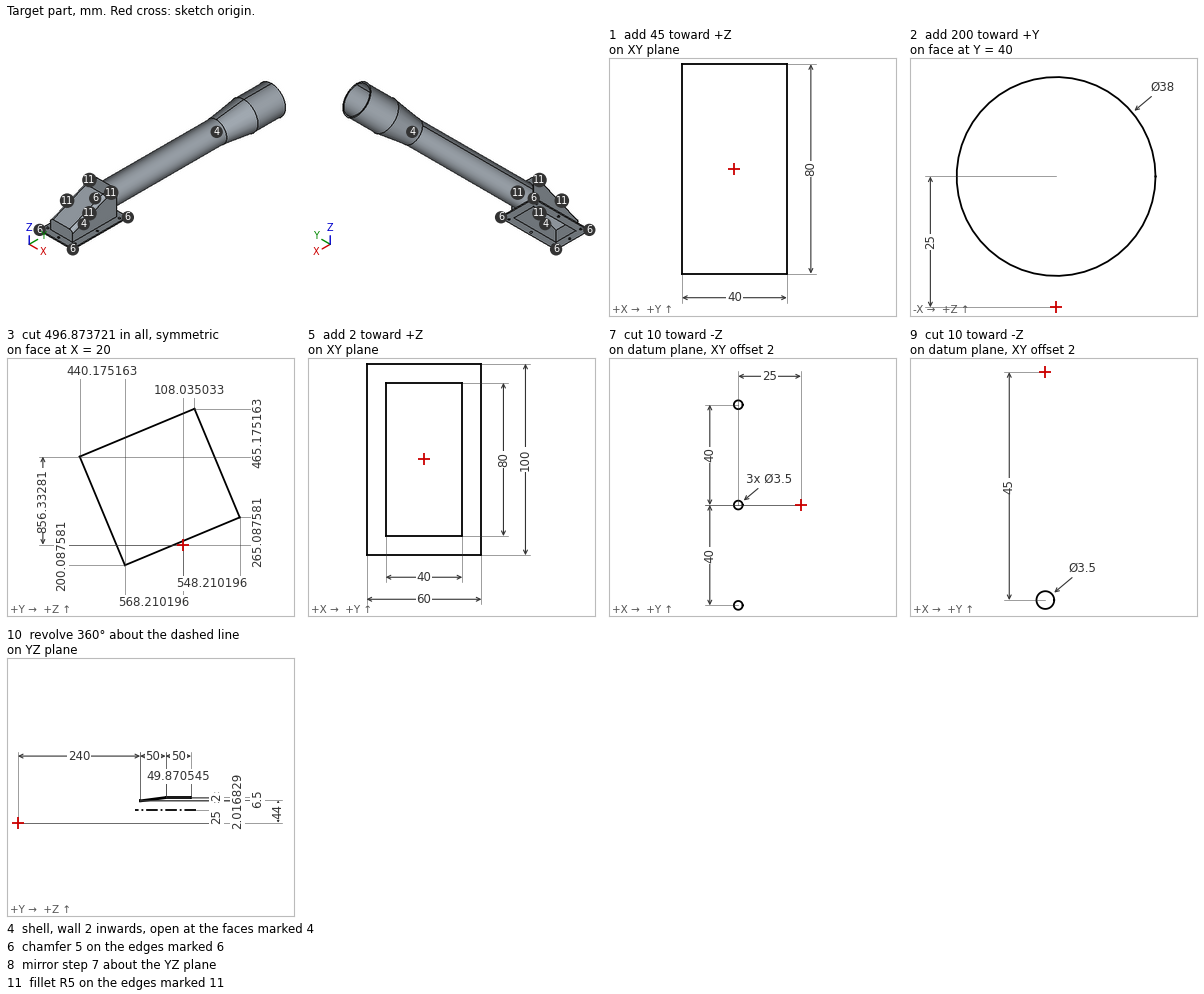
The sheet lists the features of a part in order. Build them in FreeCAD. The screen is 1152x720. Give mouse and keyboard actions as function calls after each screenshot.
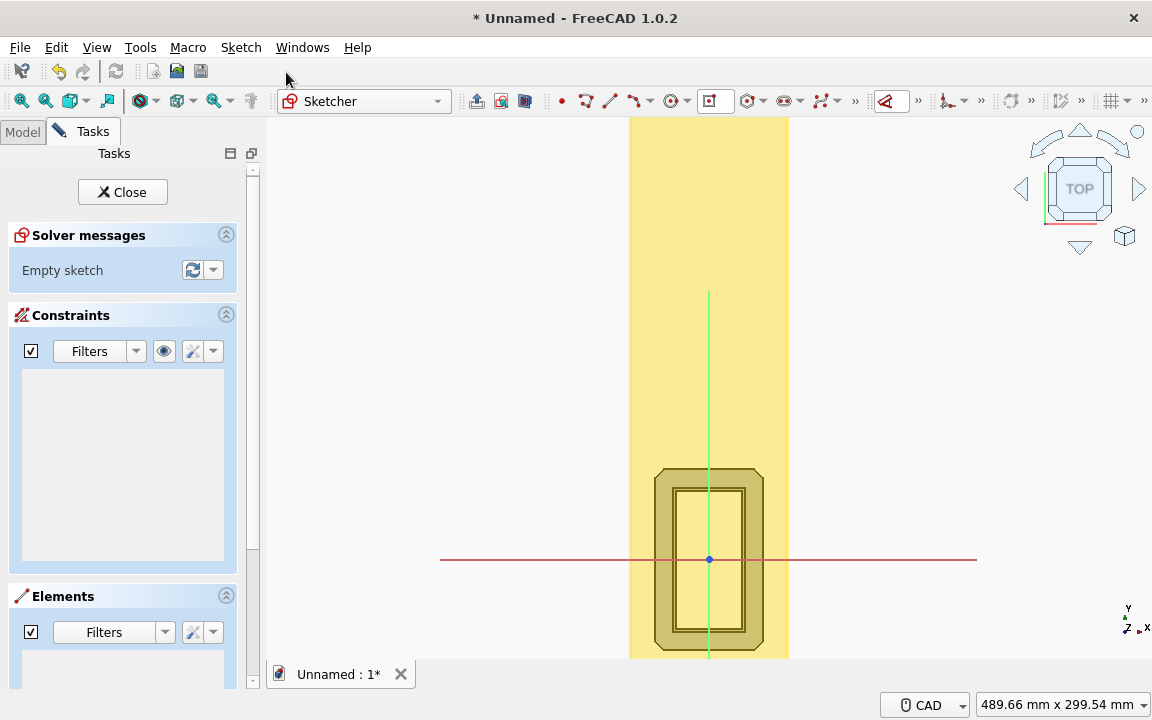
scroll(640, 388, down, 5)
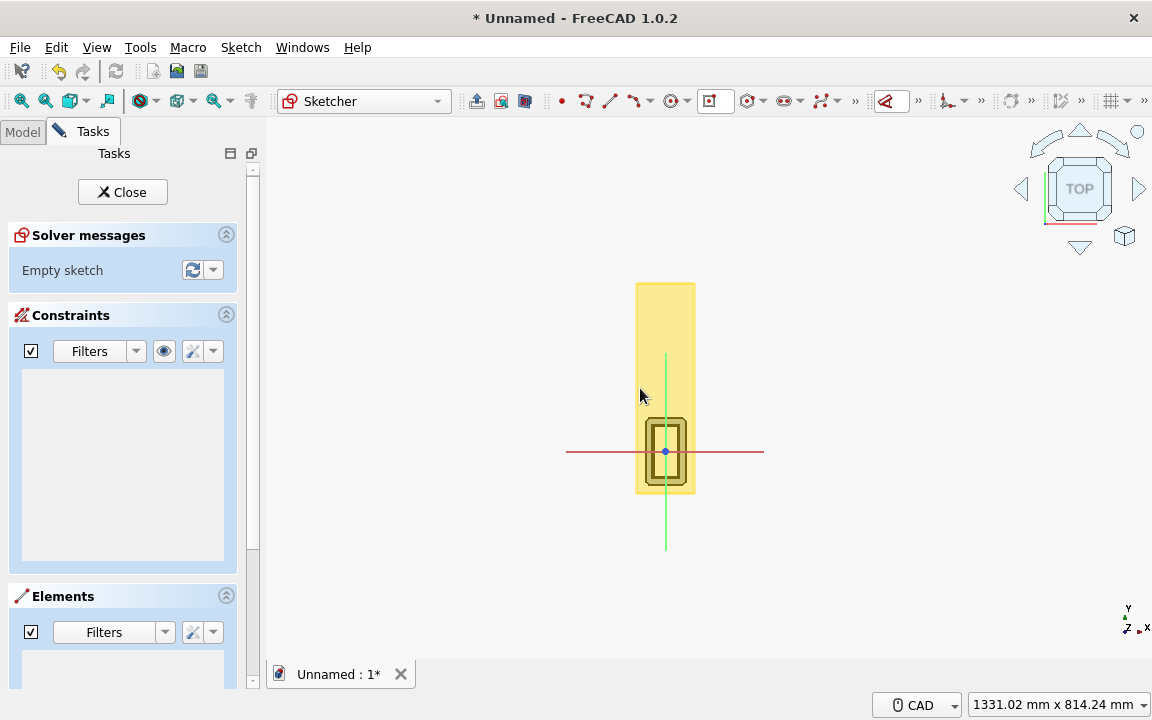
scroll(660, 464, up, 9)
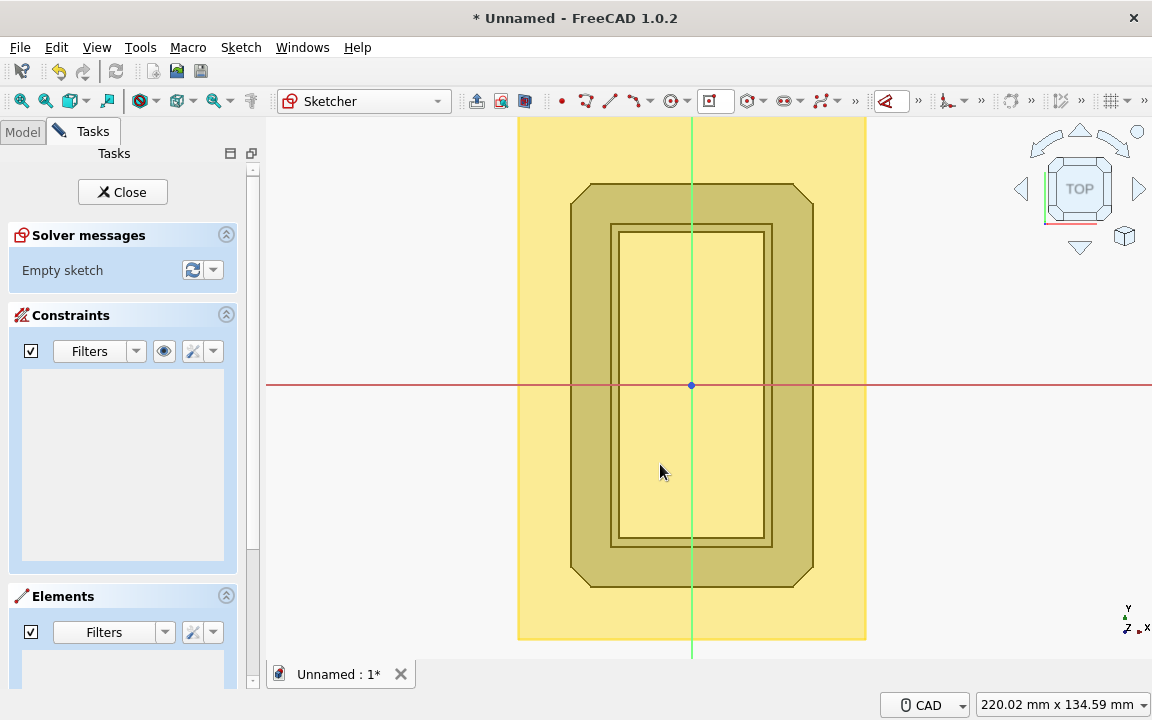
key(g)
key(c)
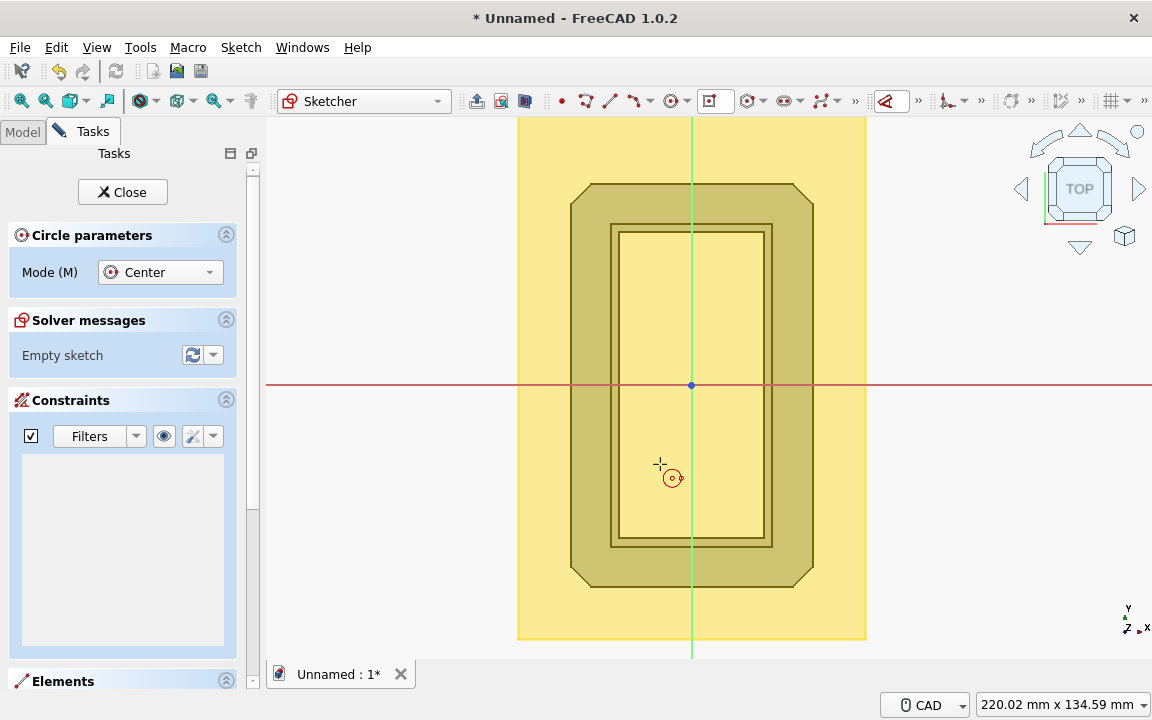
scroll(591, 385, up, 6)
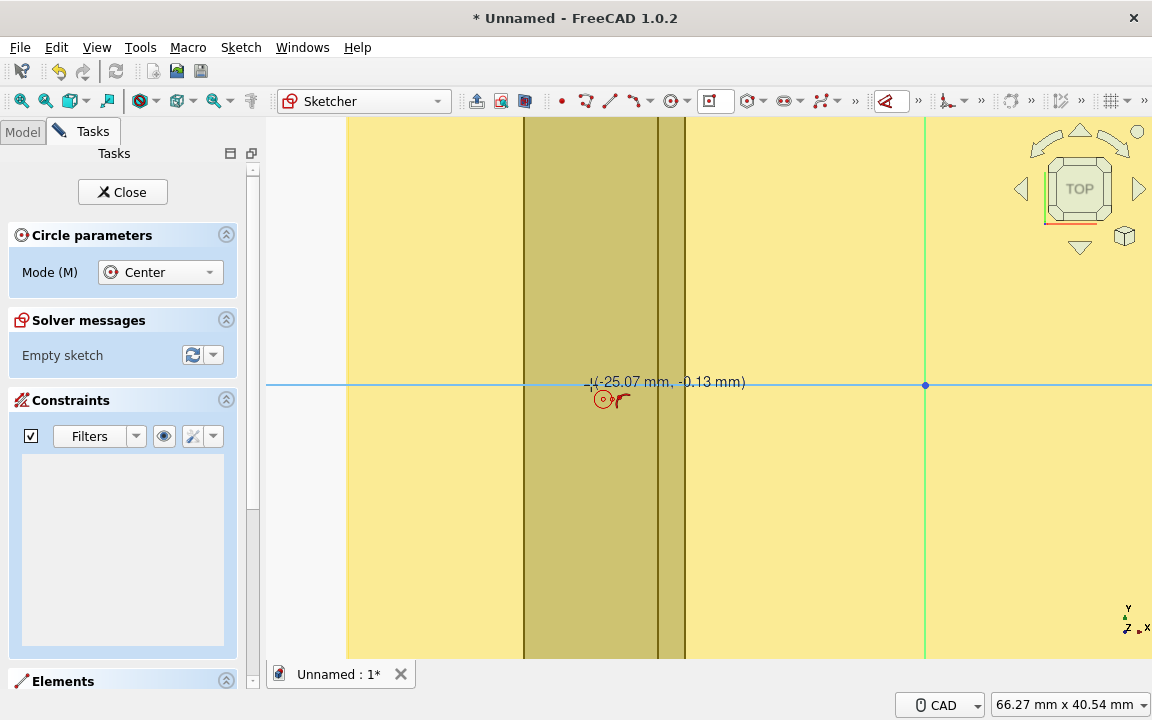
click(591, 385)
move(608, 369)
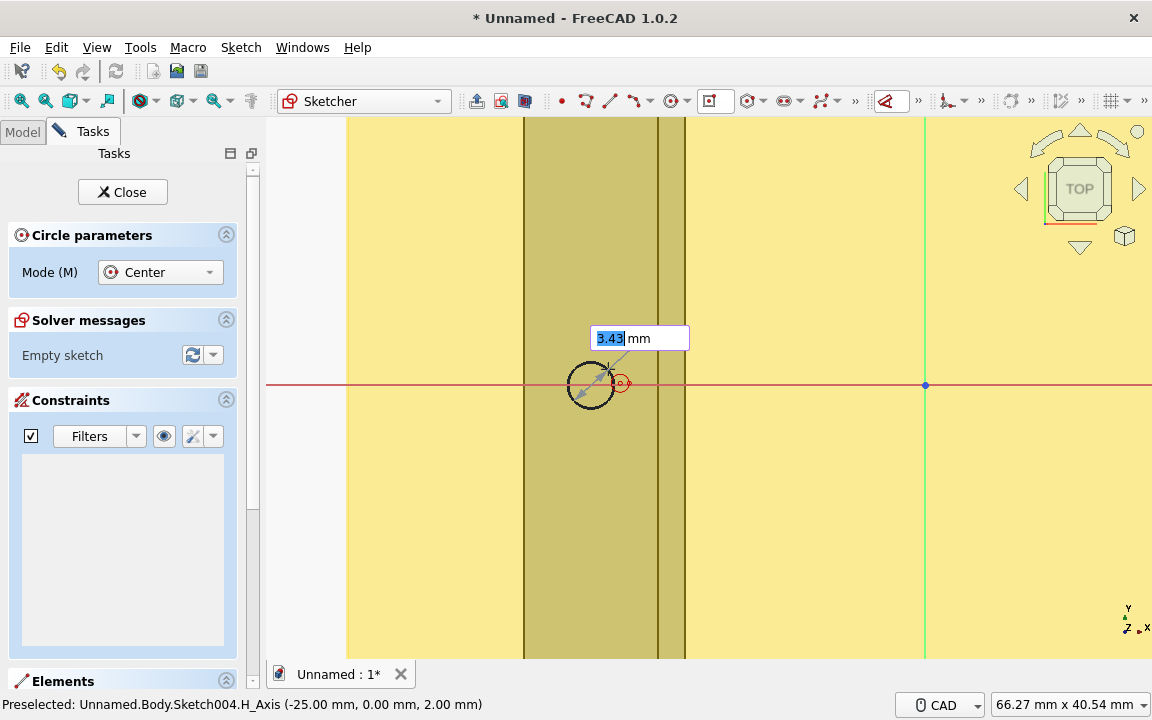
text(3.5)
key(Return)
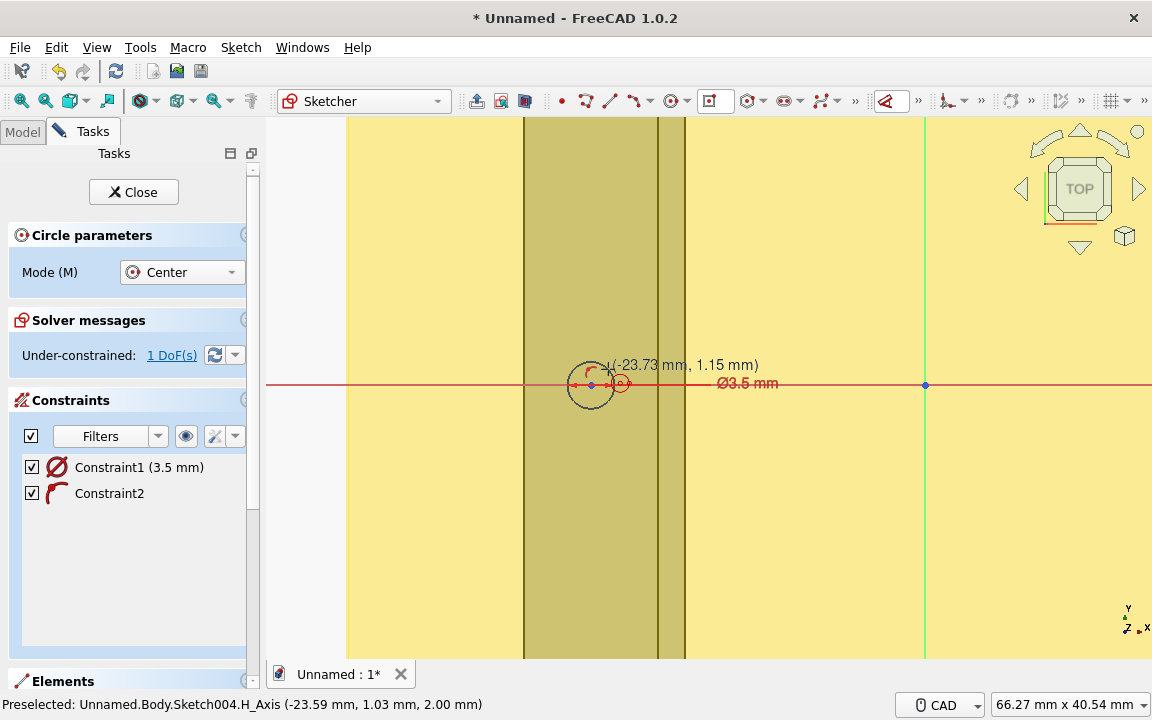
scroll(595, 389, down, 6)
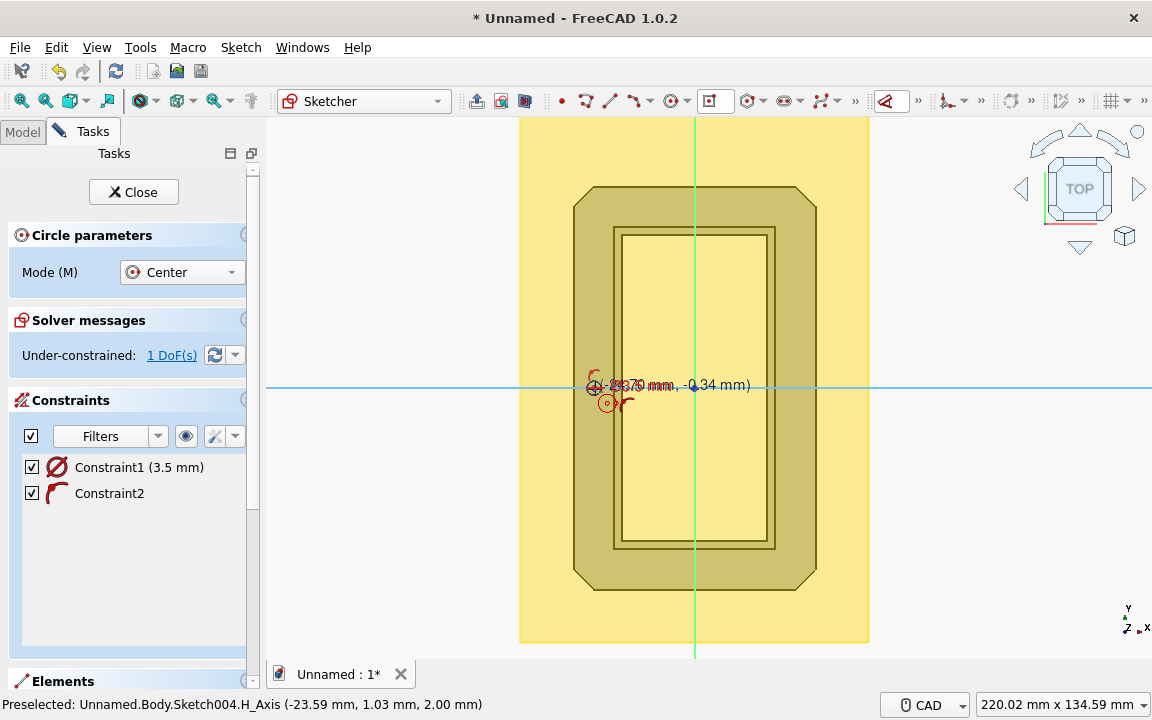
scroll(594, 227, up, 6)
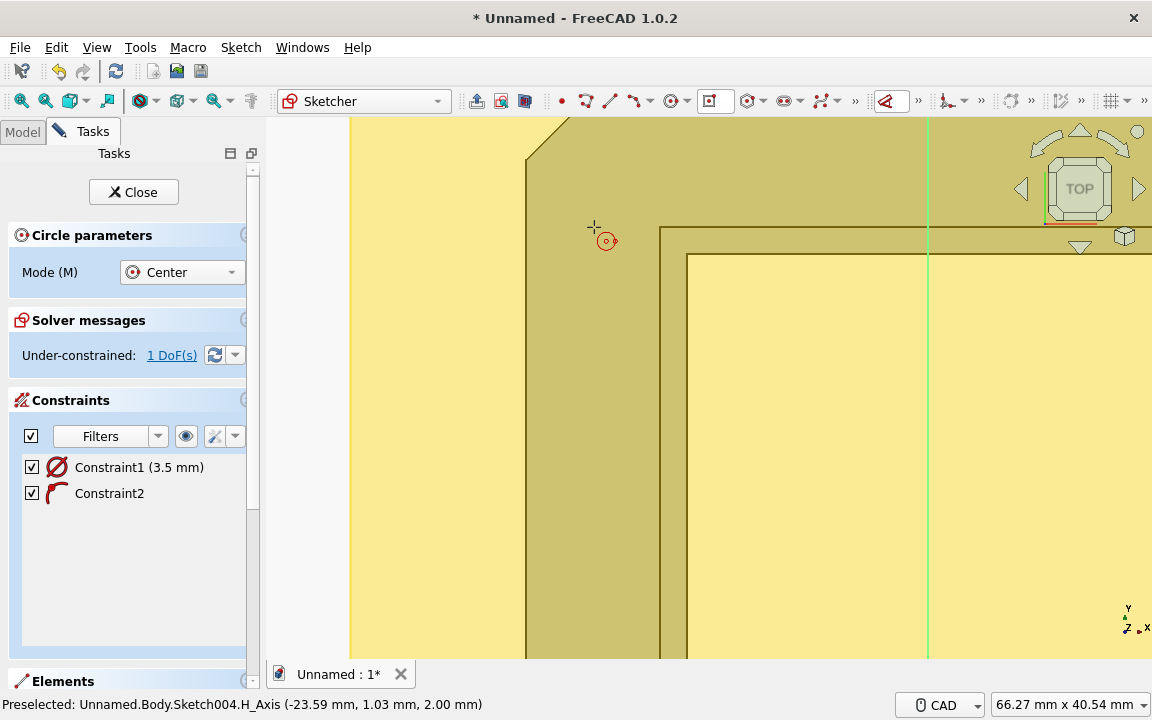
click(593, 227)
move(610, 211)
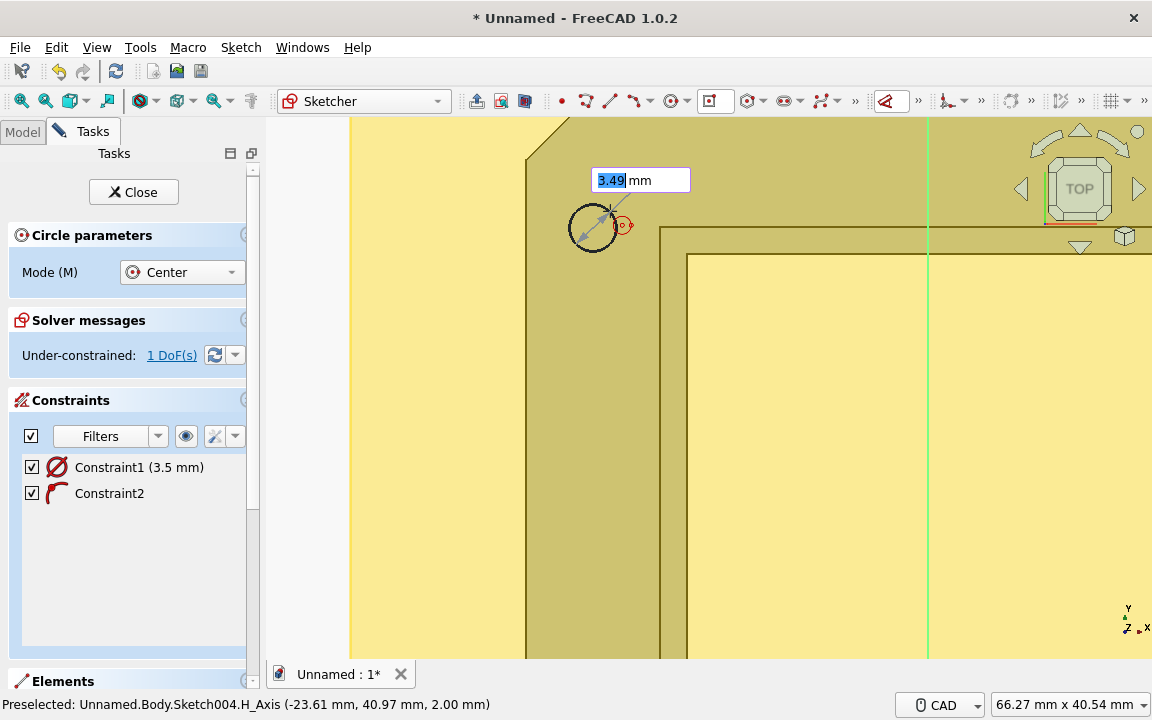
text(3.5)
key(Return)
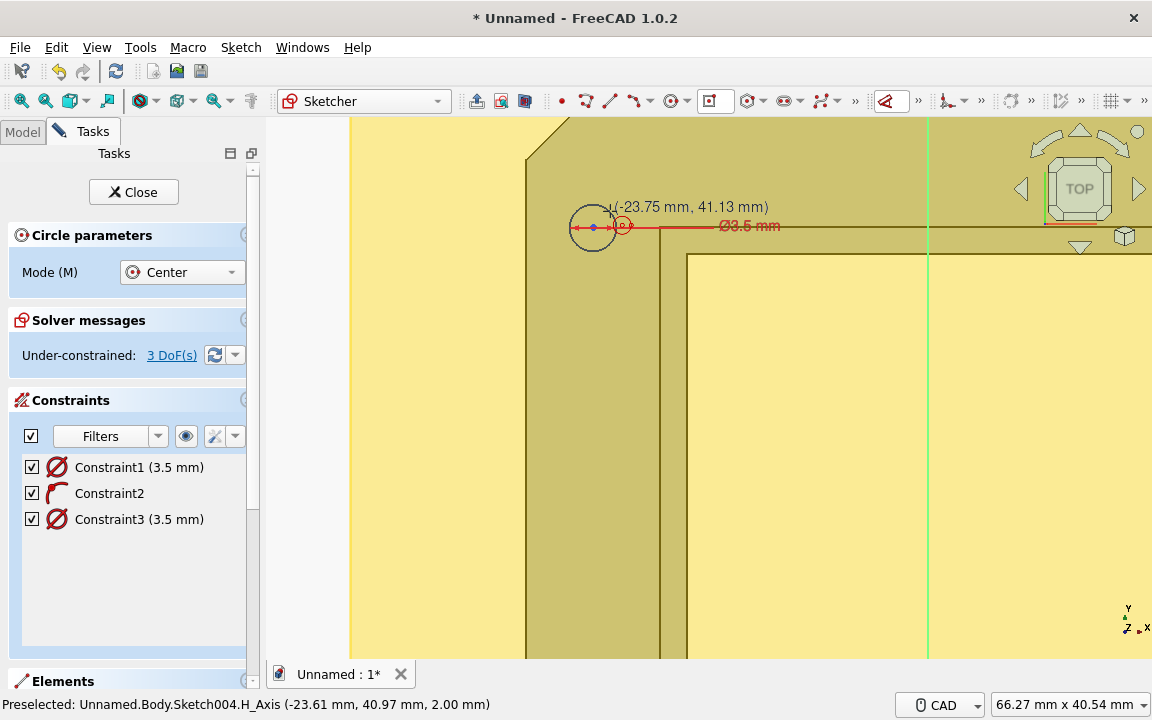
scroll(594, 227, down, 6)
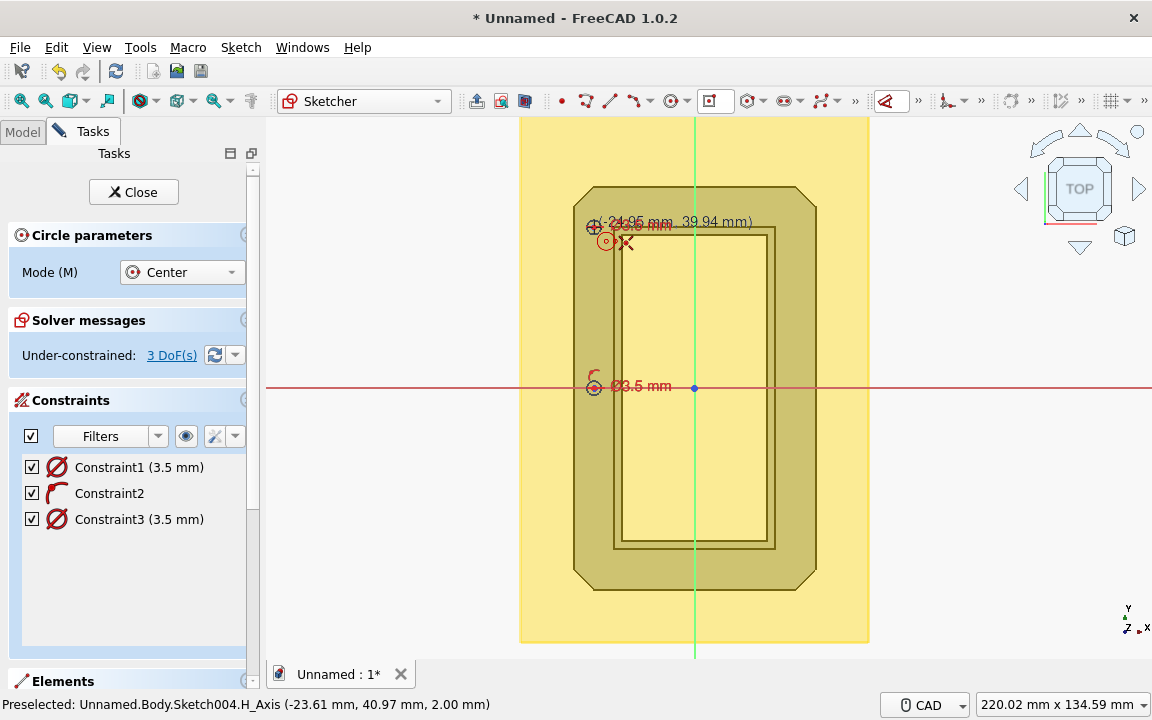
scroll(594, 549, up, 6)